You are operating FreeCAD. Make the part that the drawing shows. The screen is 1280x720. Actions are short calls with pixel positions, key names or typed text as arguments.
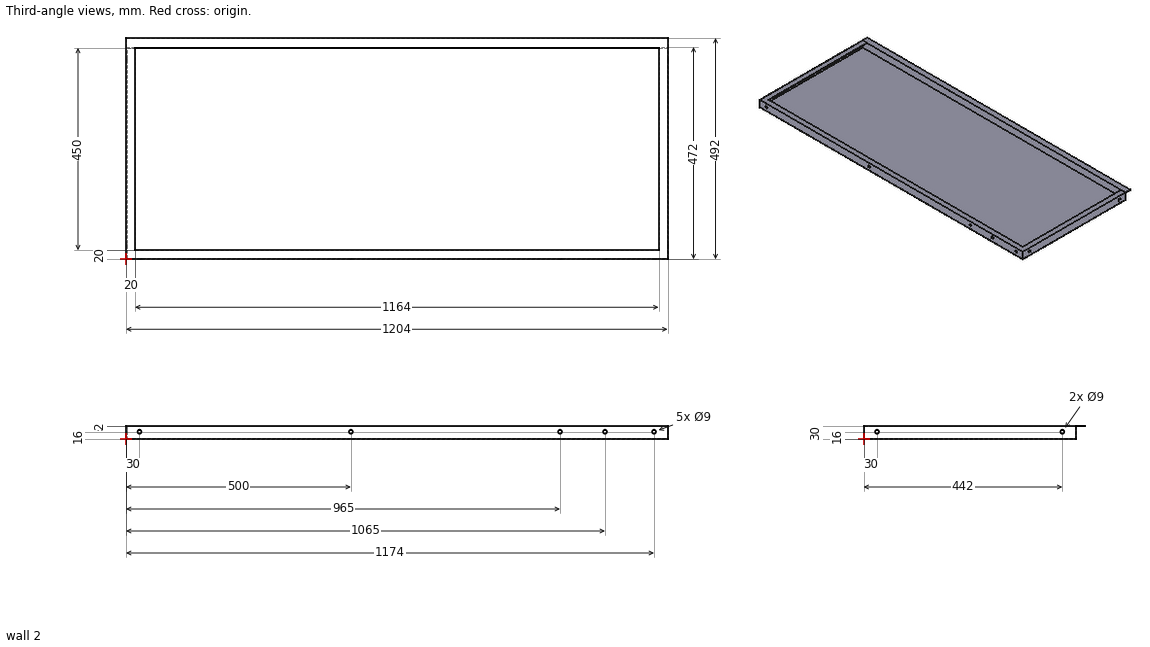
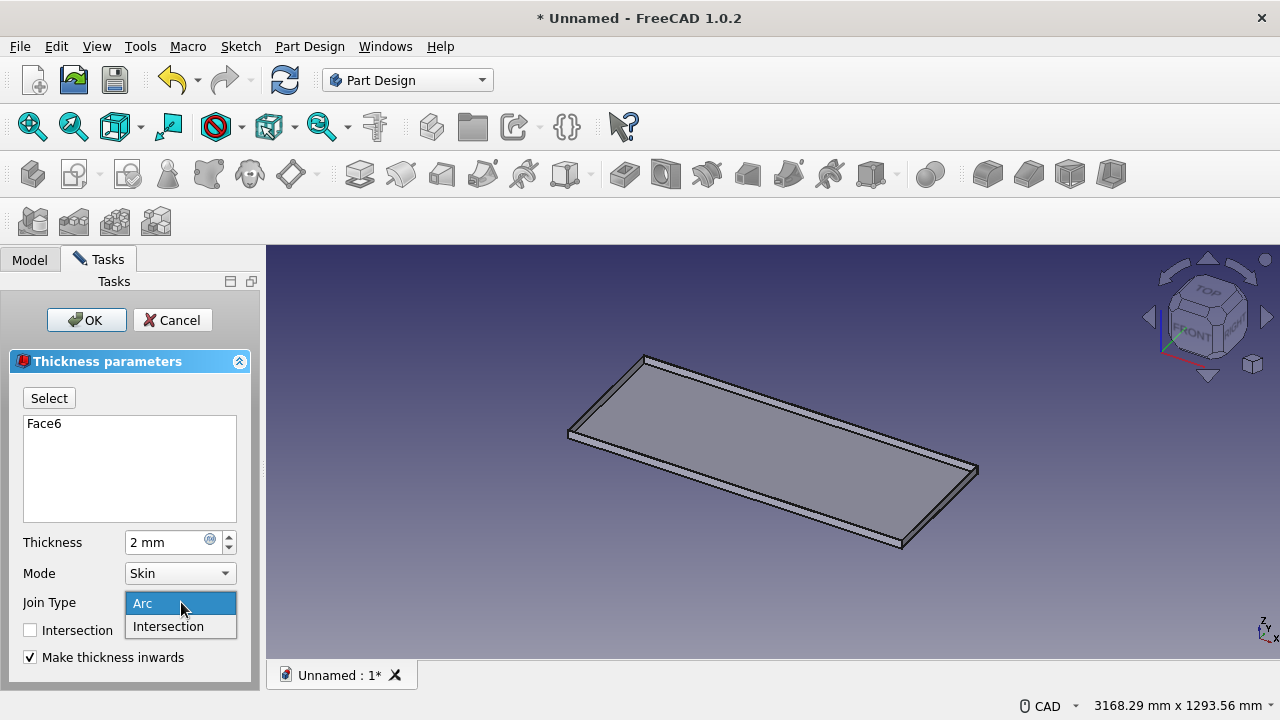
click(179, 626)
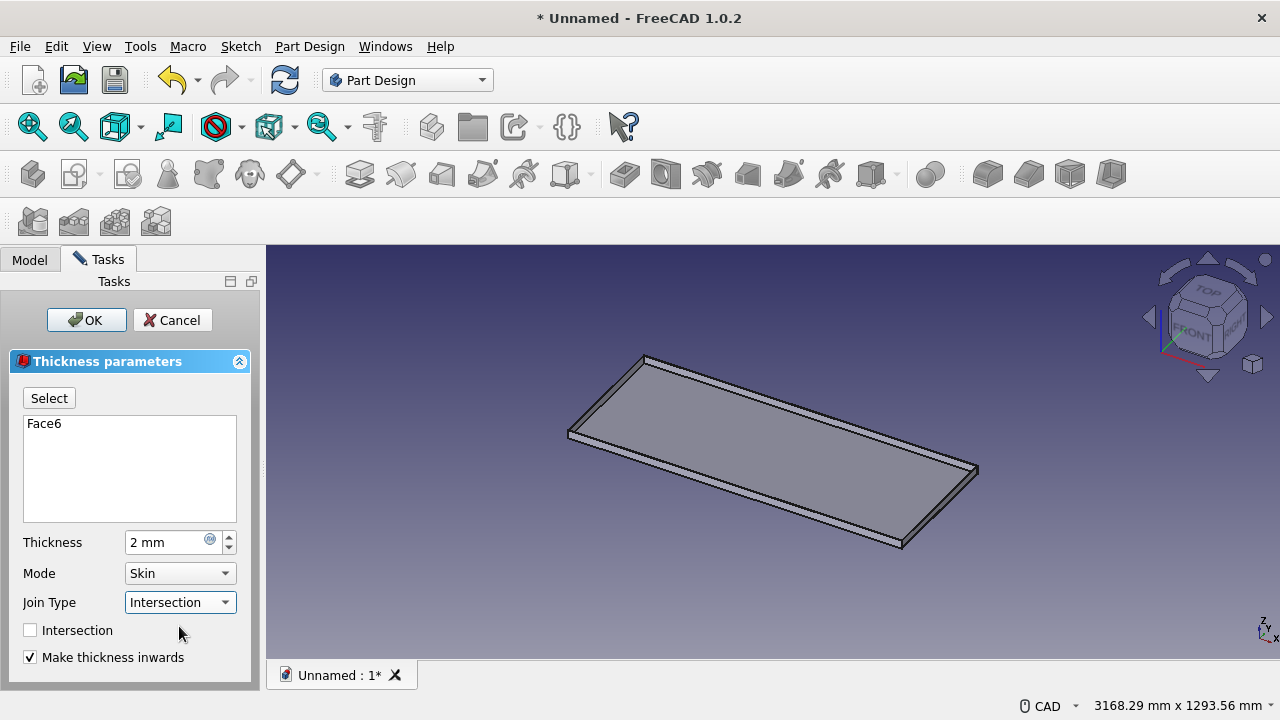
click(87, 320)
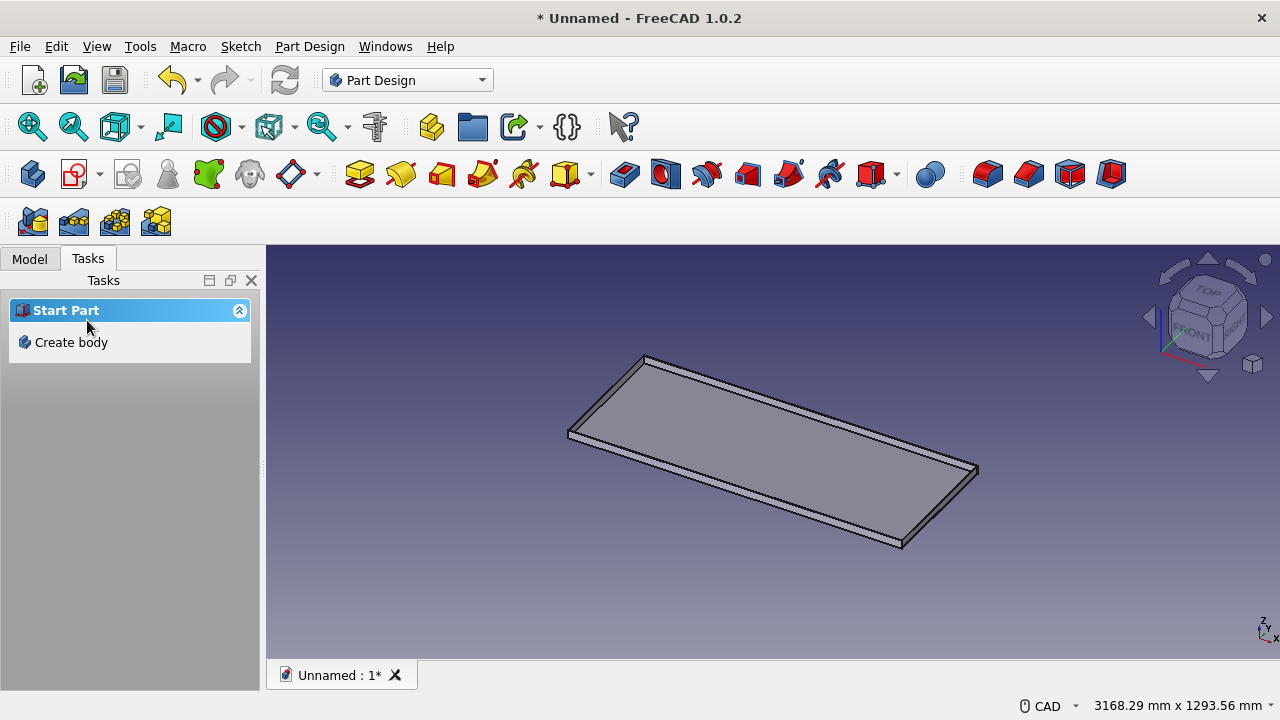
scroll(927, 515, up, 15)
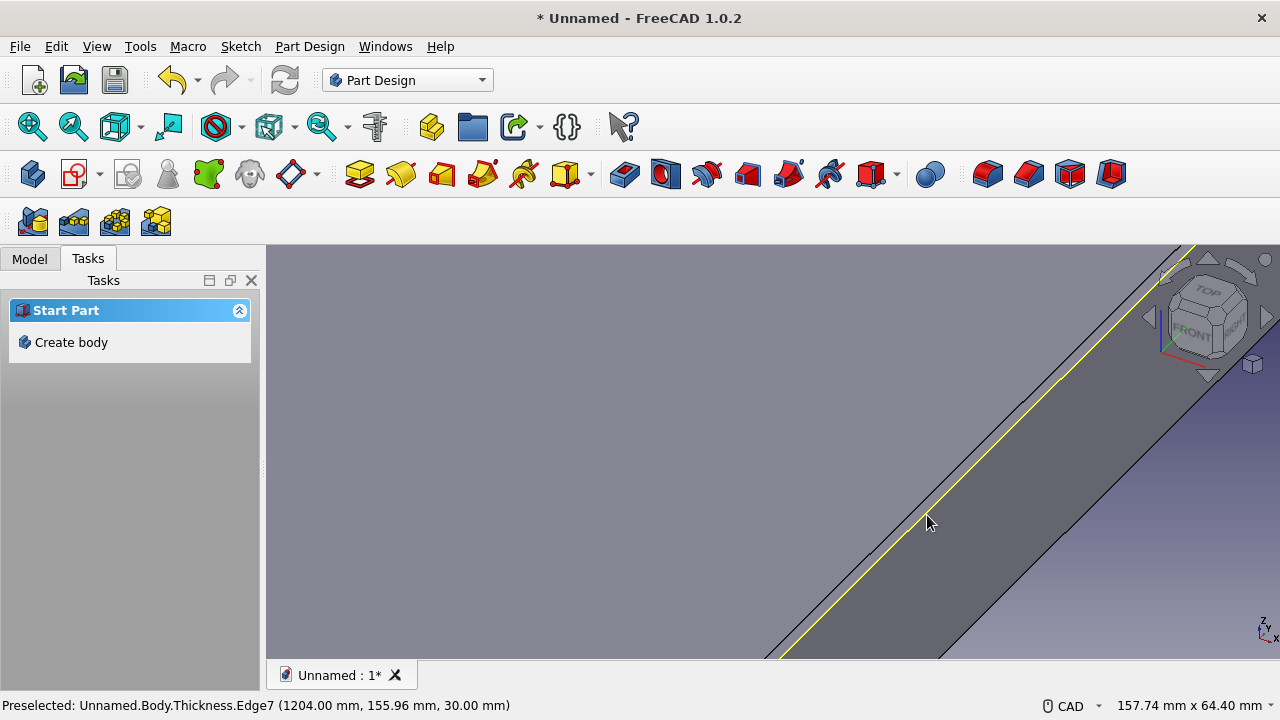
scroll(918, 515, up, 6)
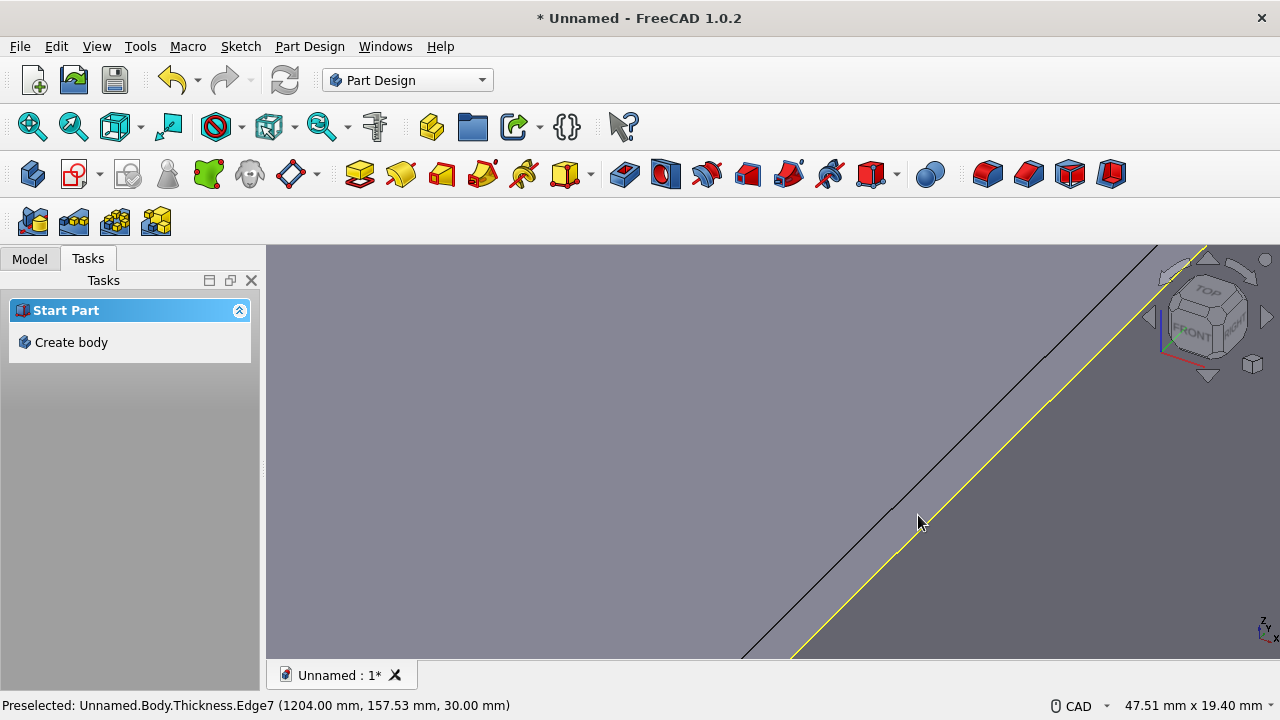
click(918, 515)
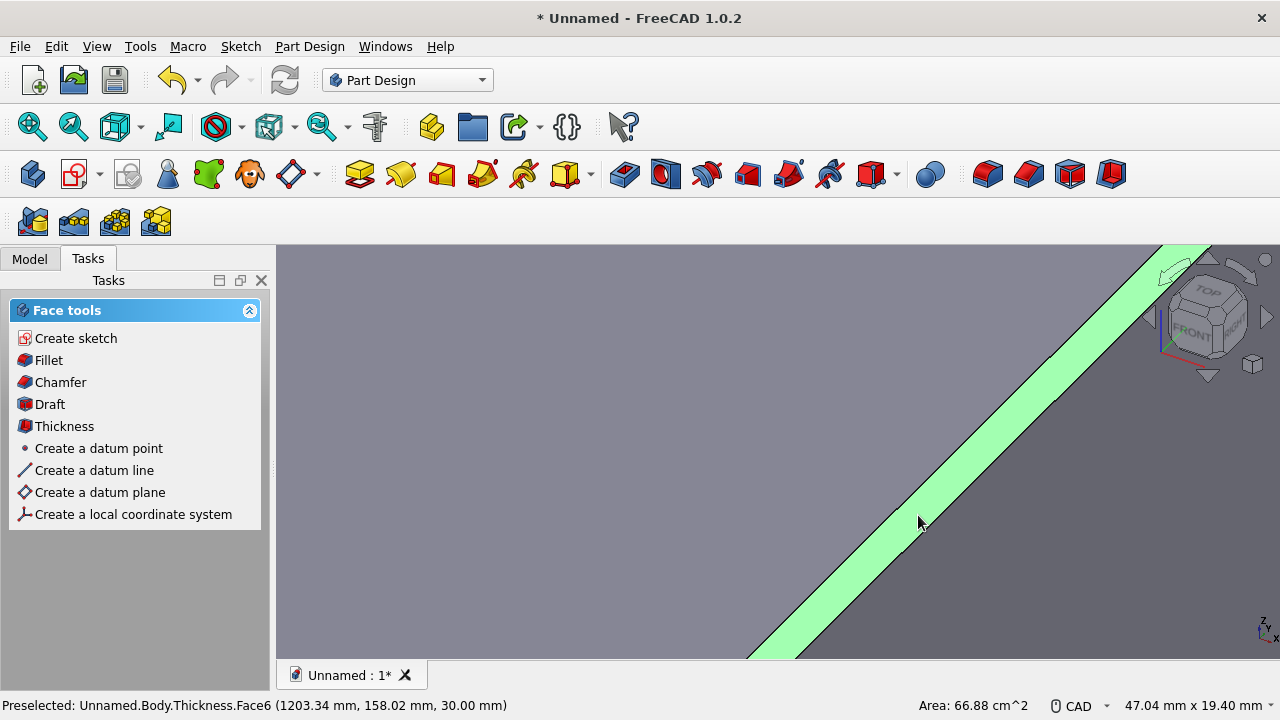
click(74, 174)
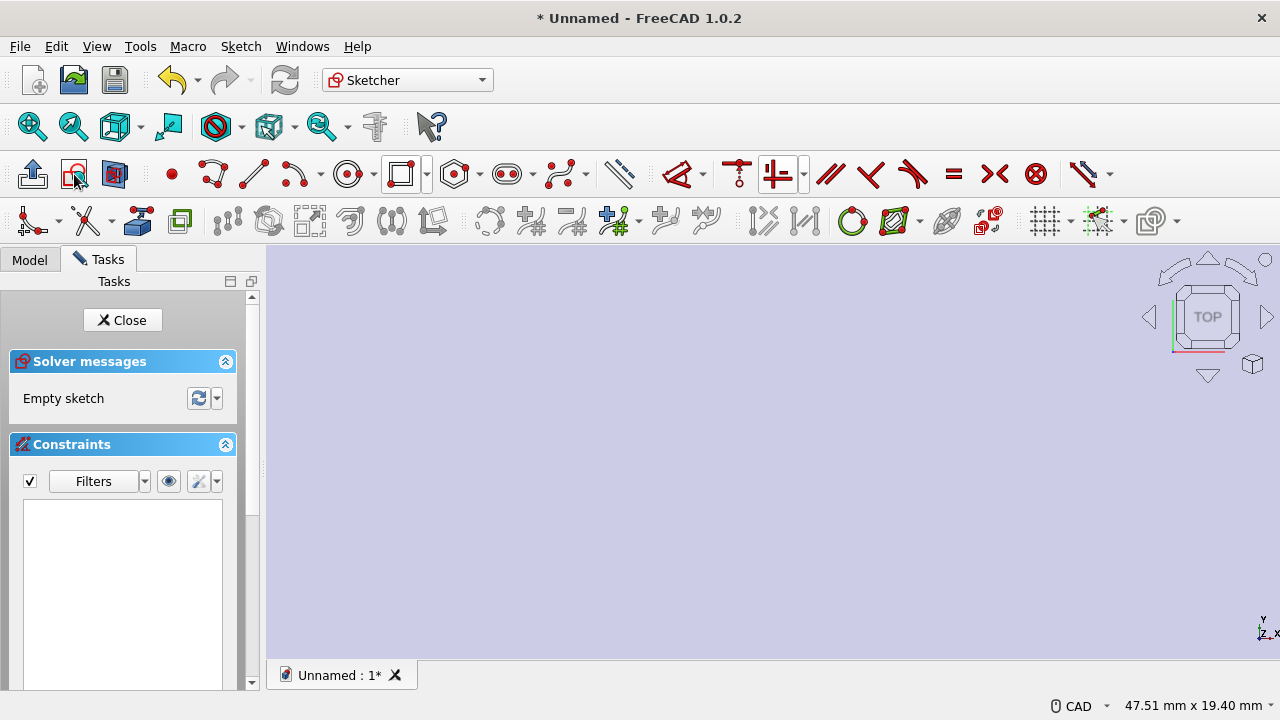
scroll(983, 374, down, 18)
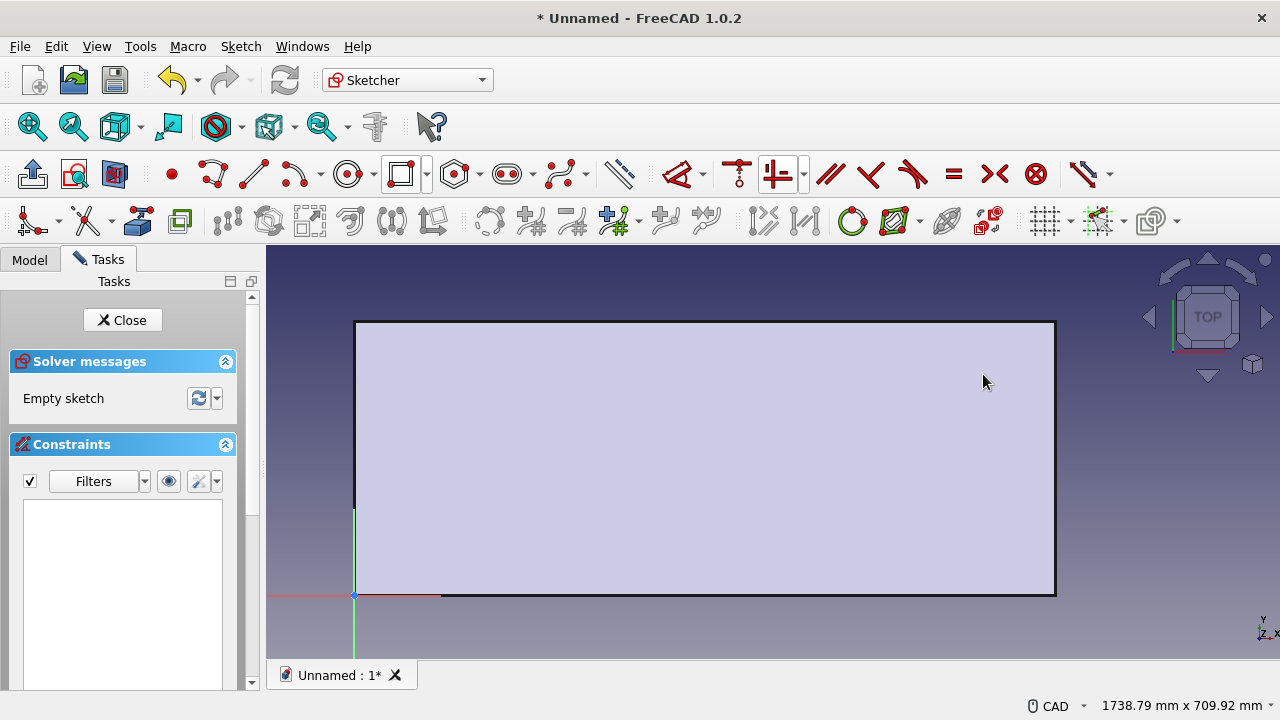
key(g)
key(r)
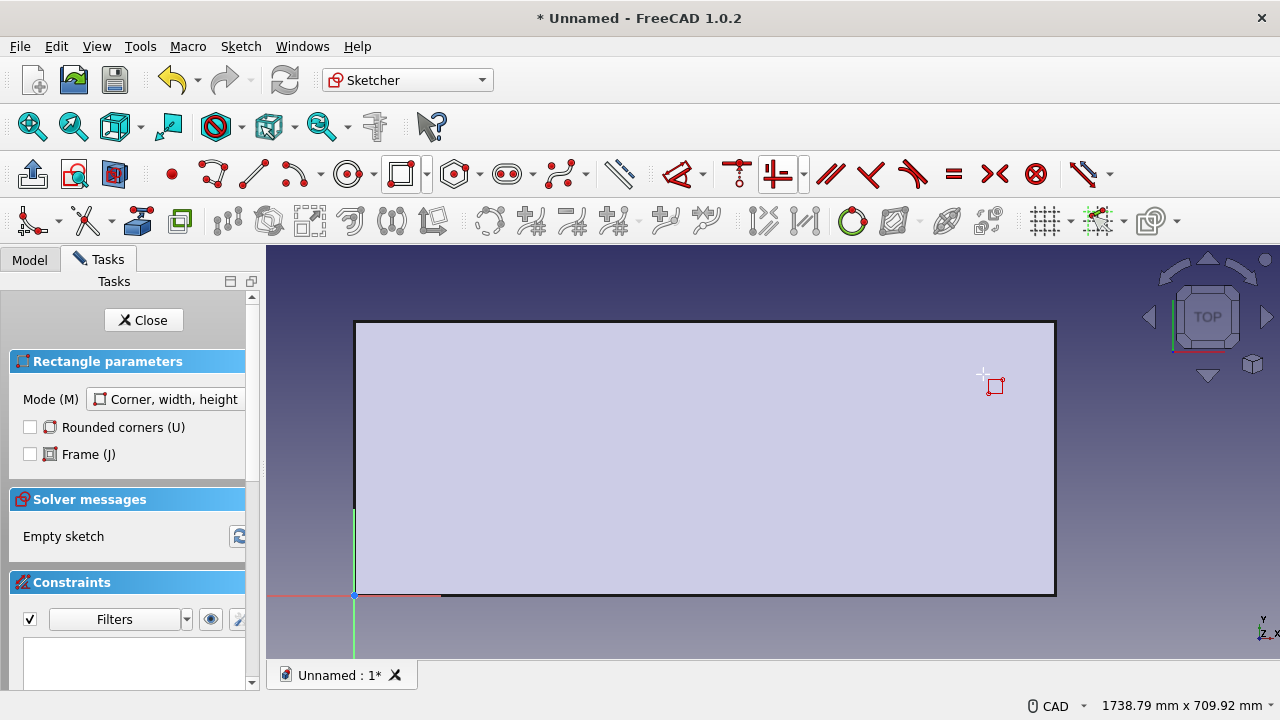
click(354, 596)
click(1056, 309)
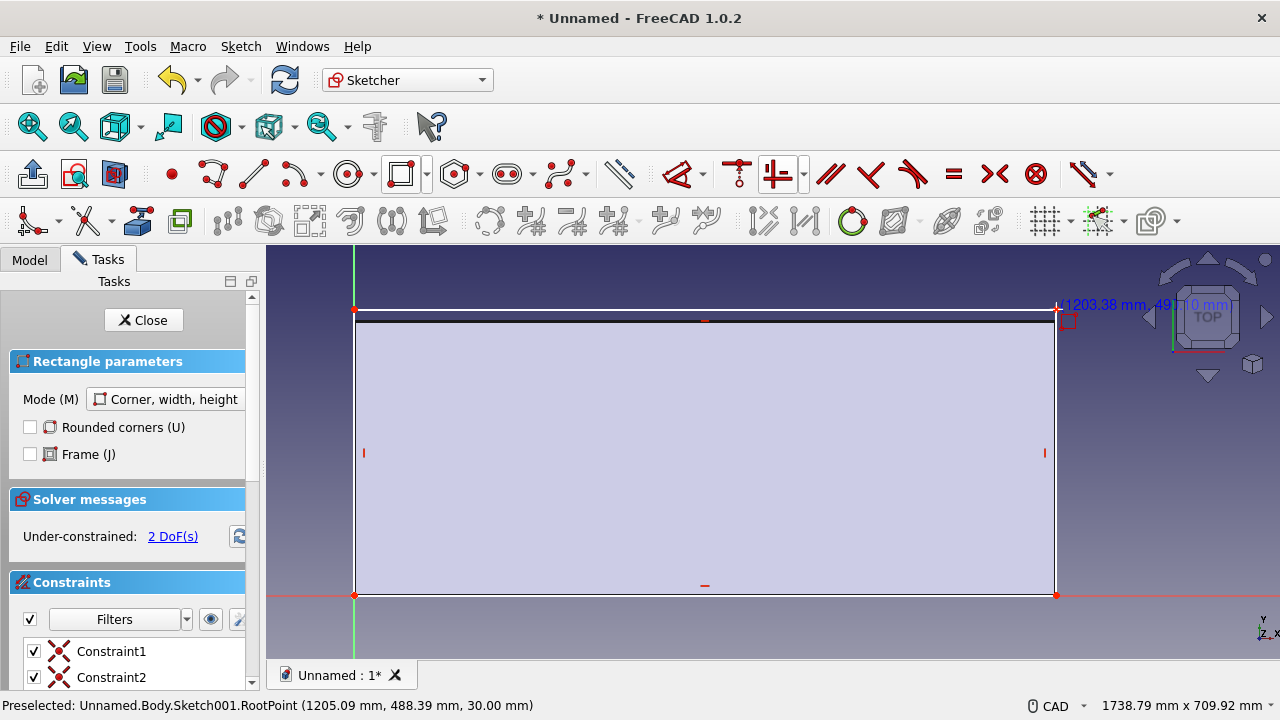
scroll(366, 322, up, 2)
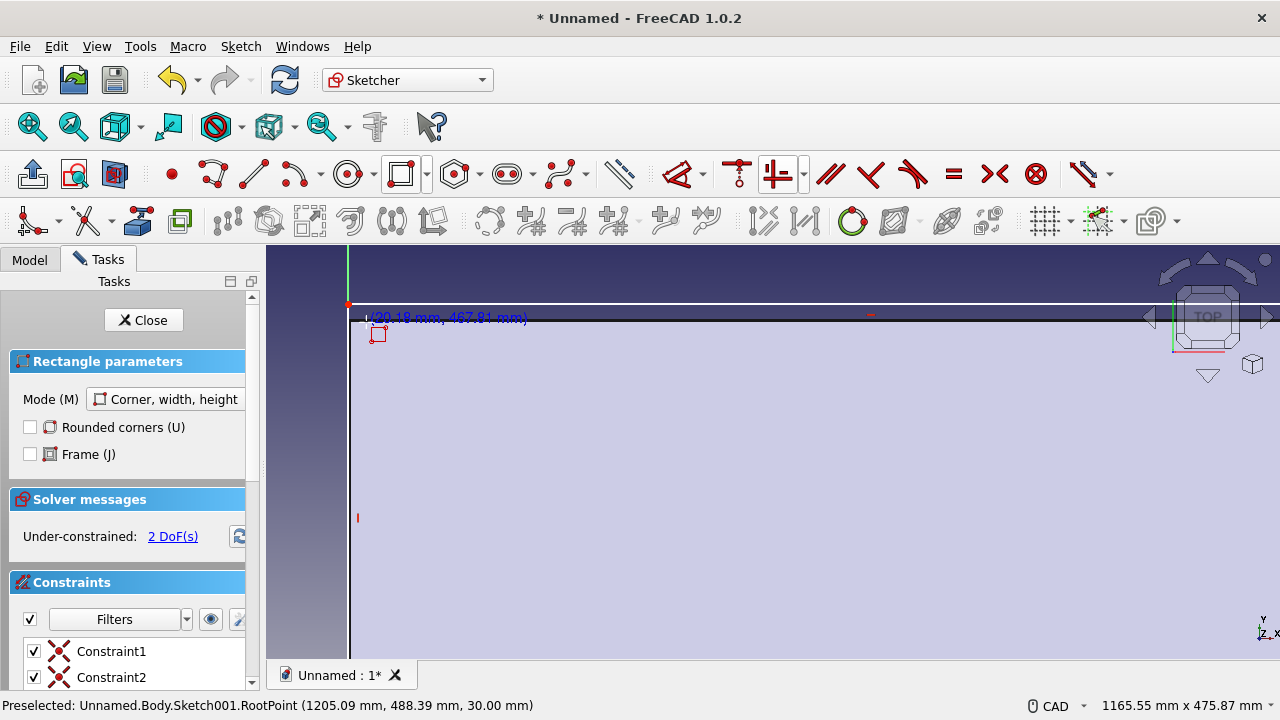
click(366, 321)